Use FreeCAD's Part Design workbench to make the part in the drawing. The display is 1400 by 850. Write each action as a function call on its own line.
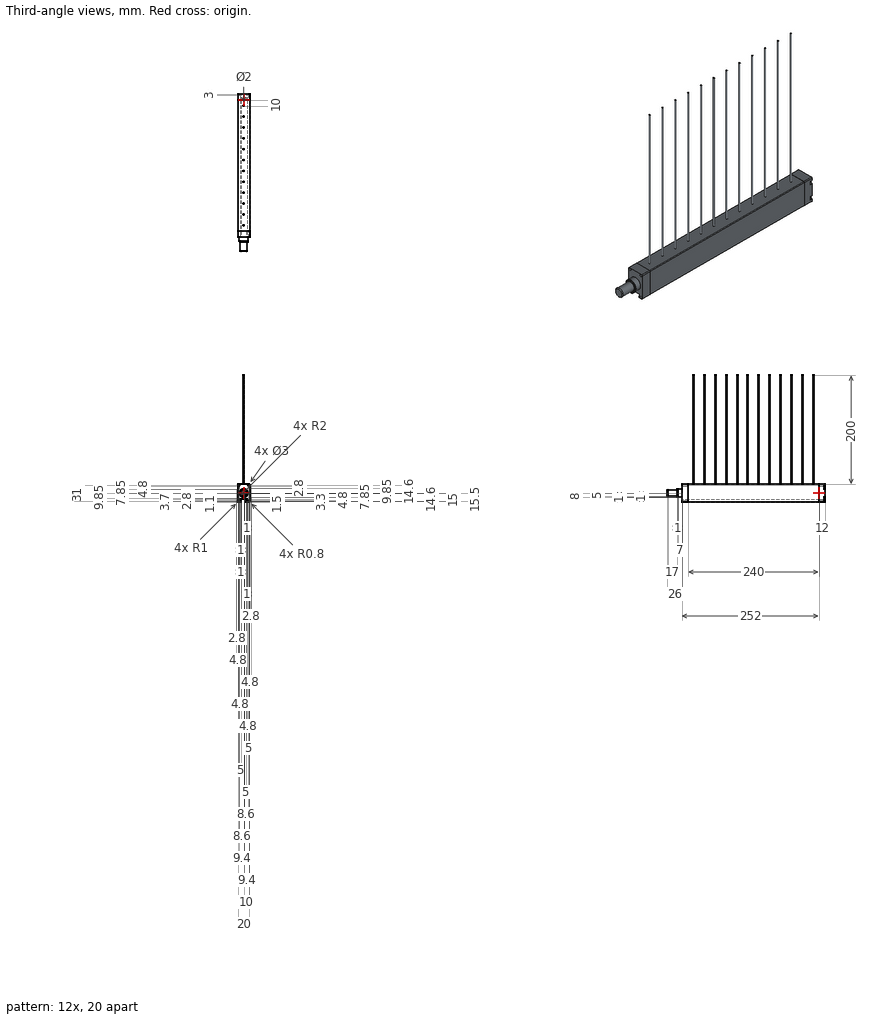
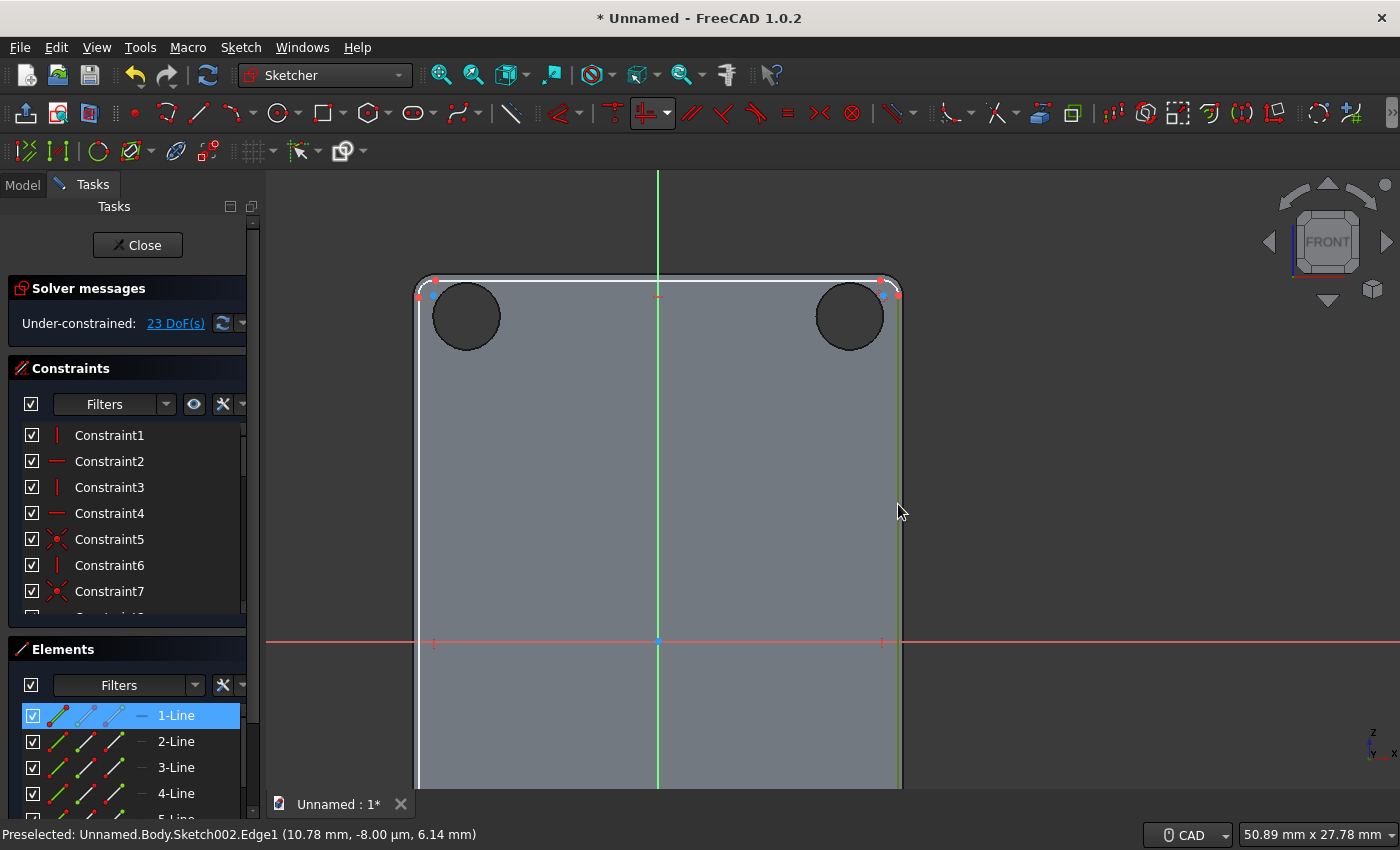
scroll(894, 282, down, 3)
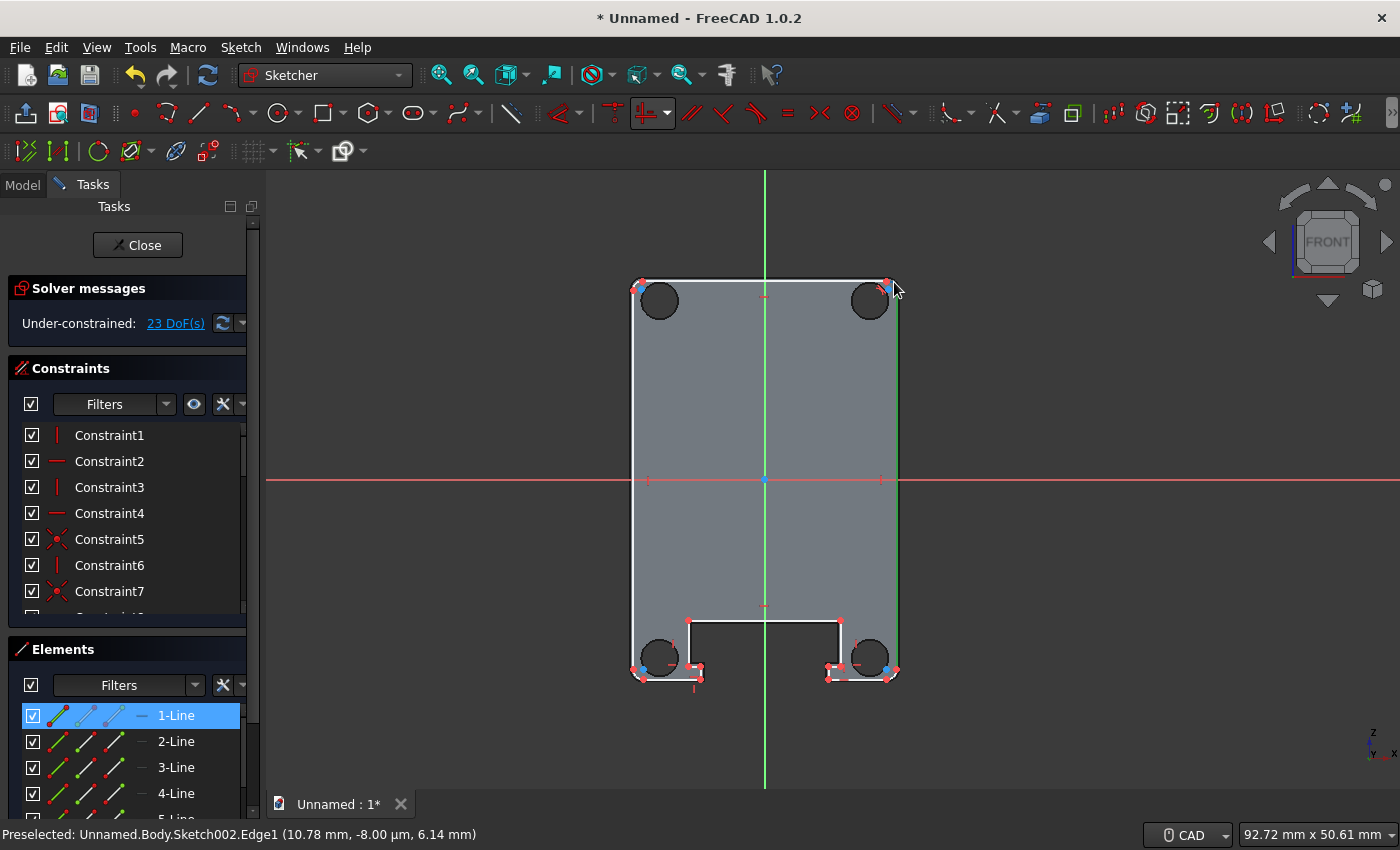
scroll(894, 677, up, 4)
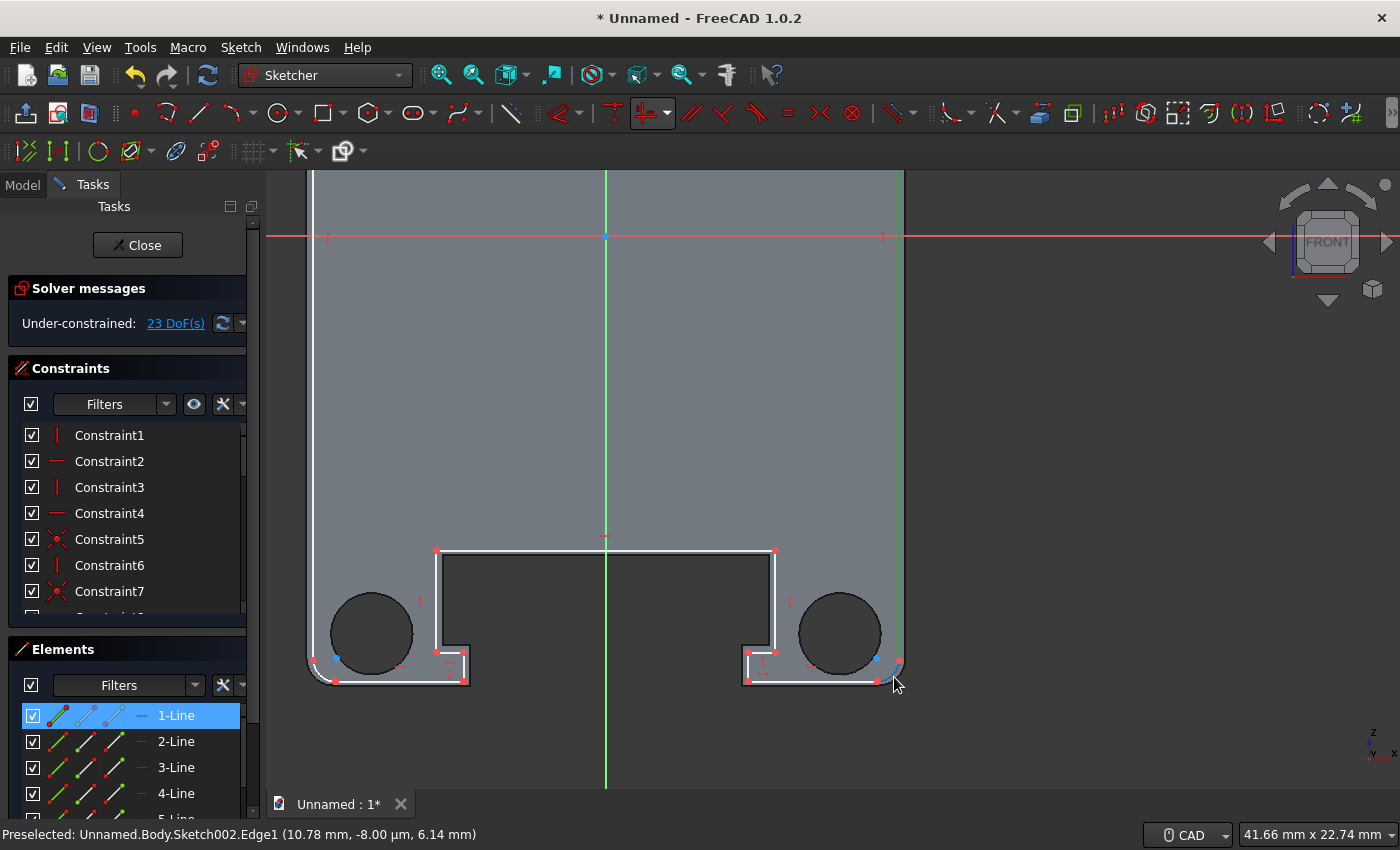
click(892, 675)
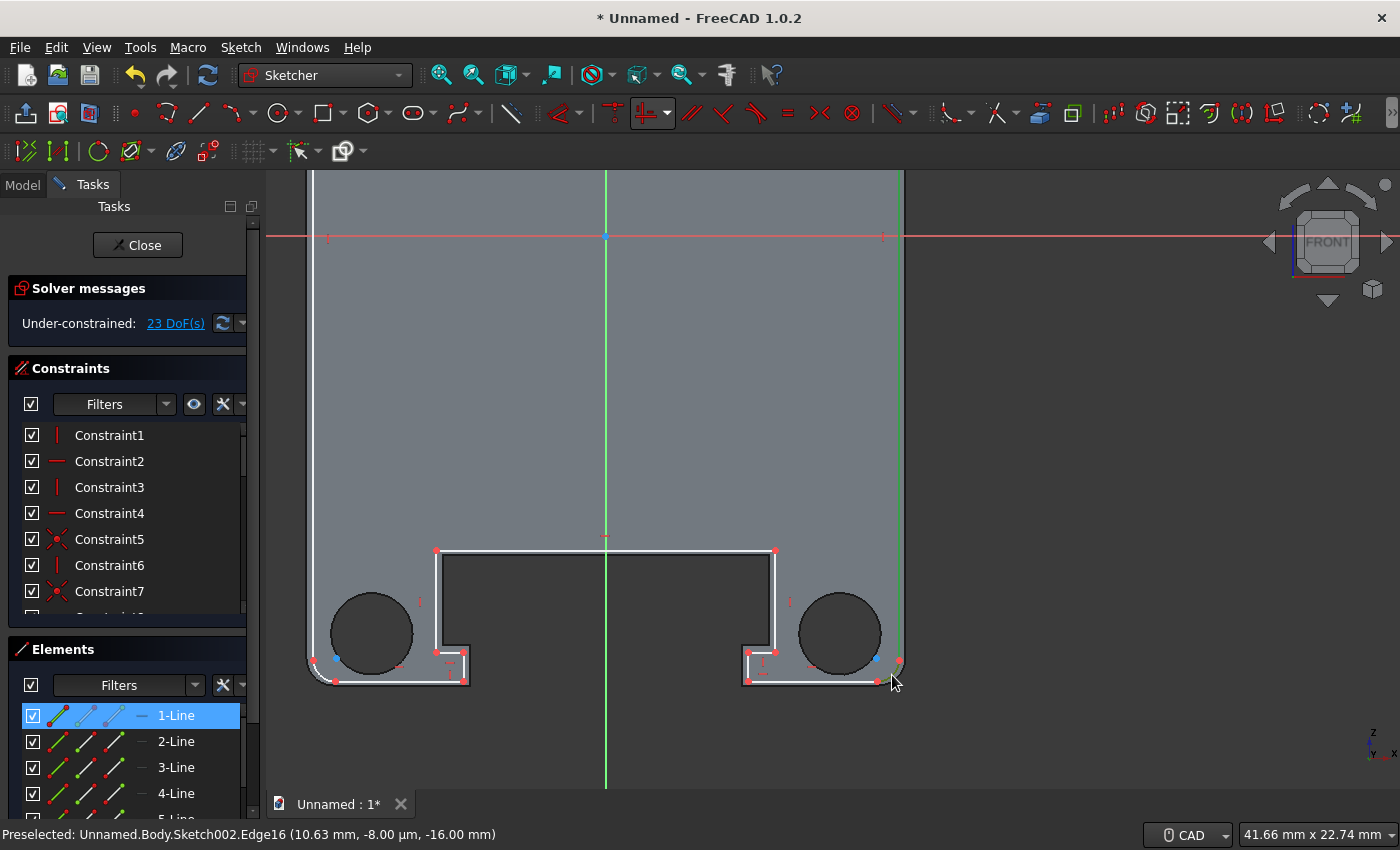
click(756, 114)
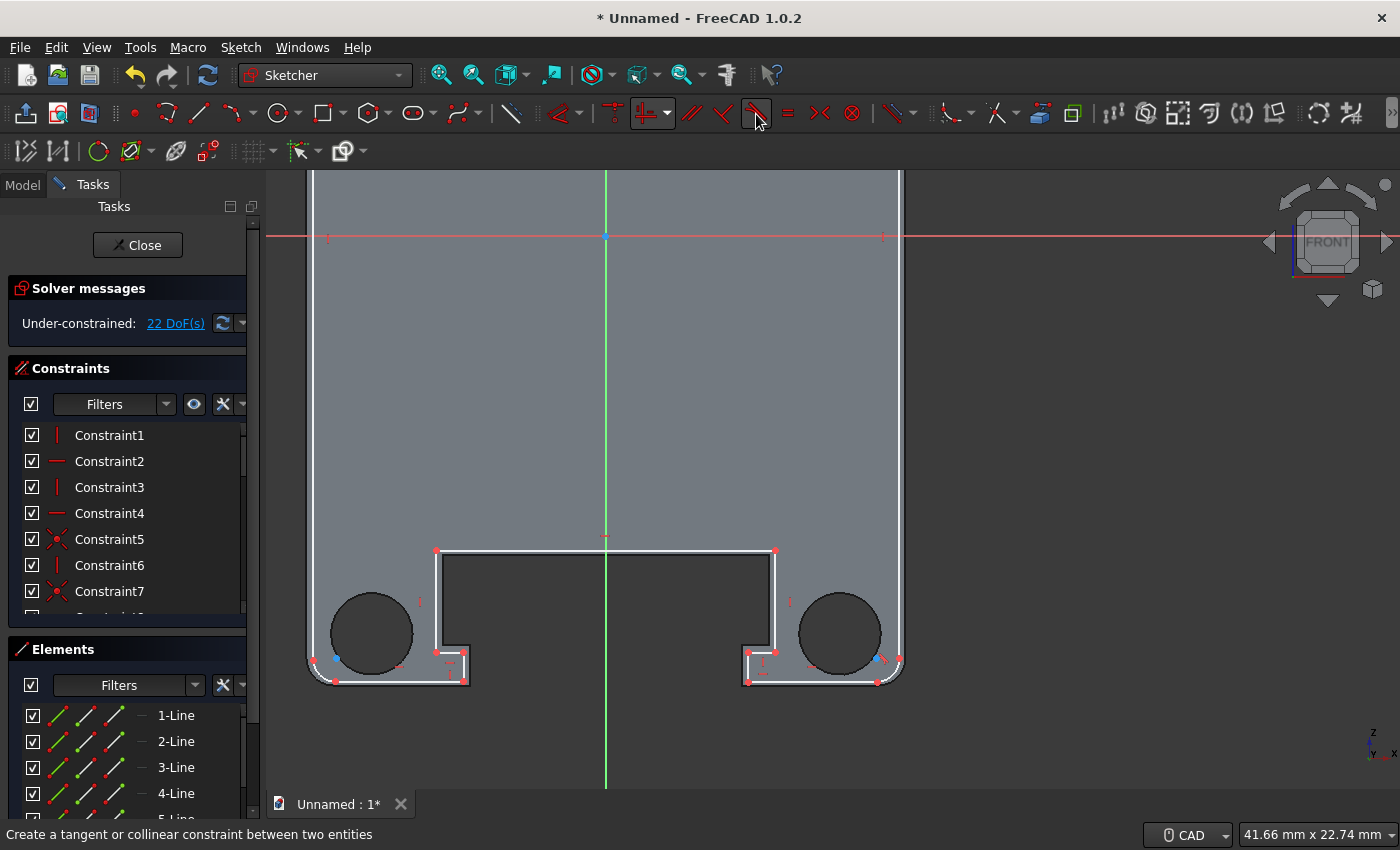
scroll(894, 678, down, 4)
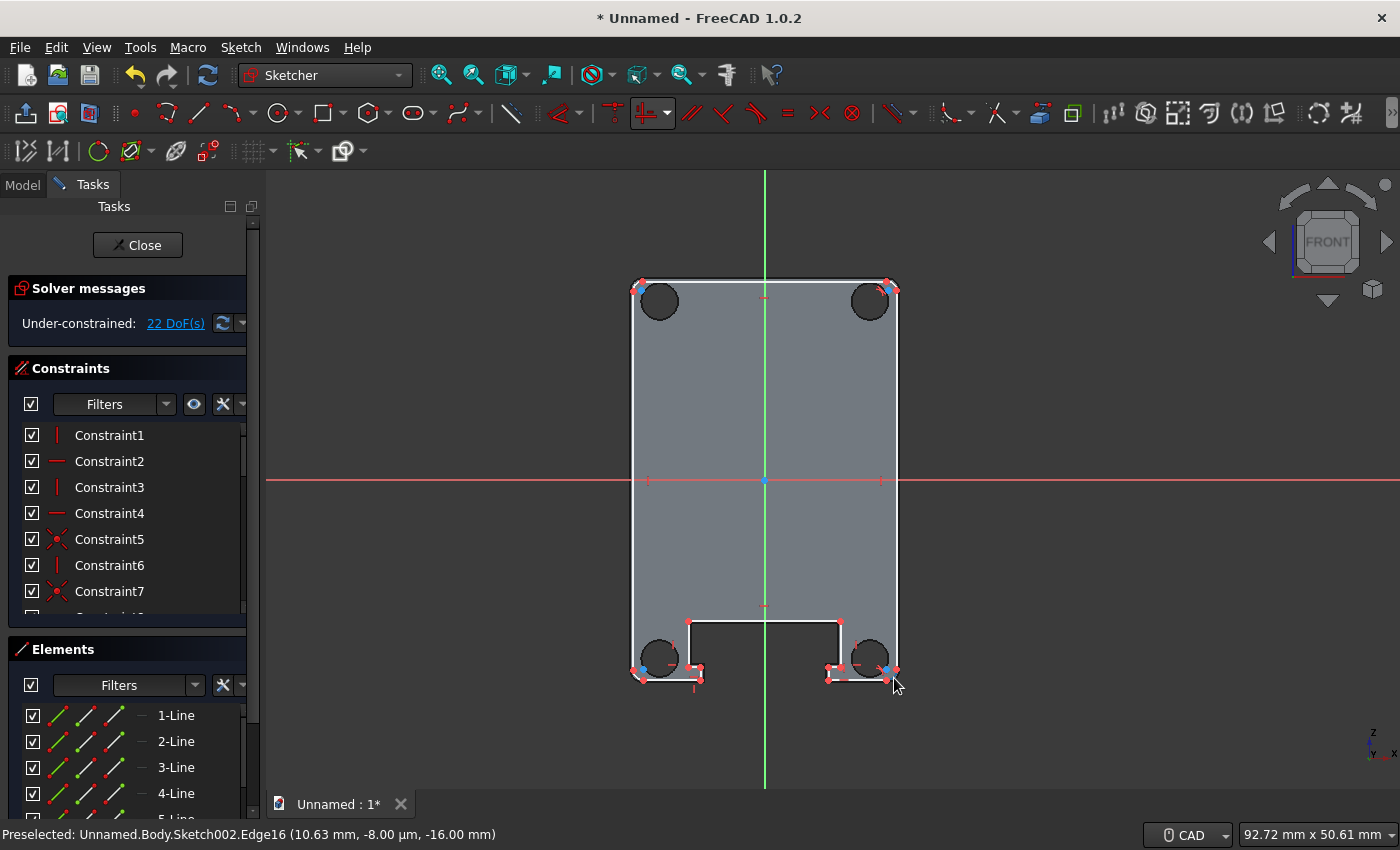
click(814, 282)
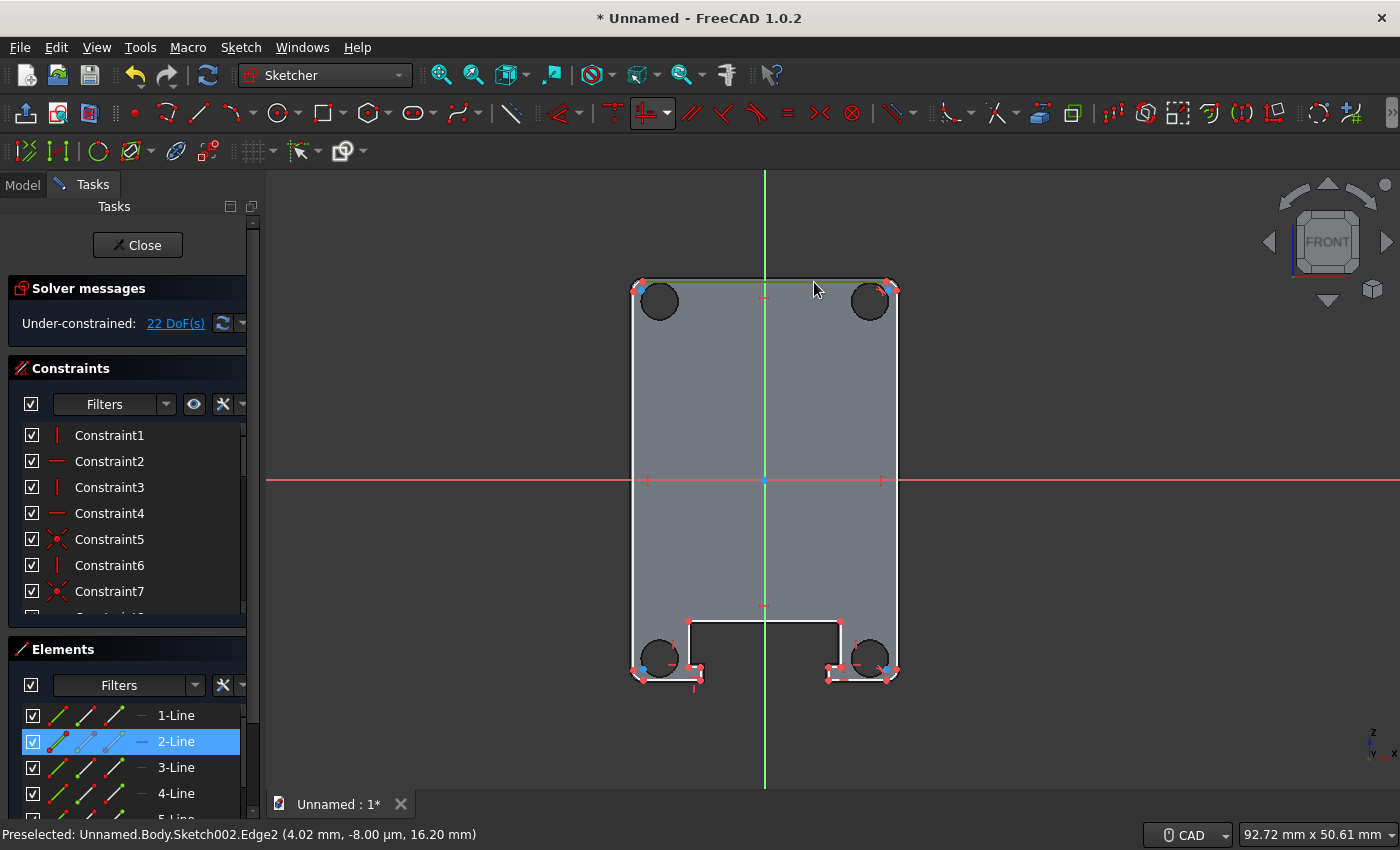
scroll(894, 284, up, 4)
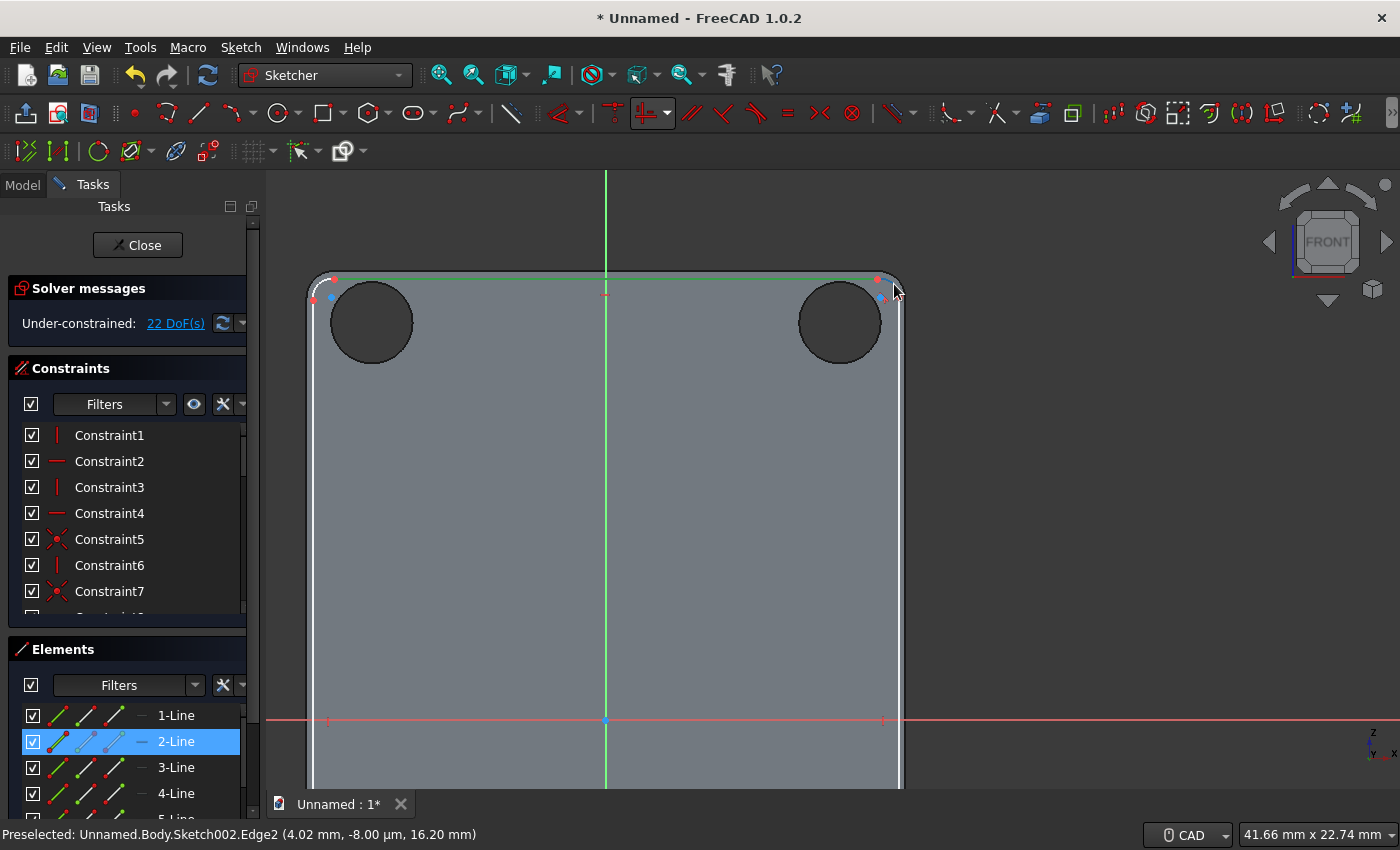
click(893, 283)